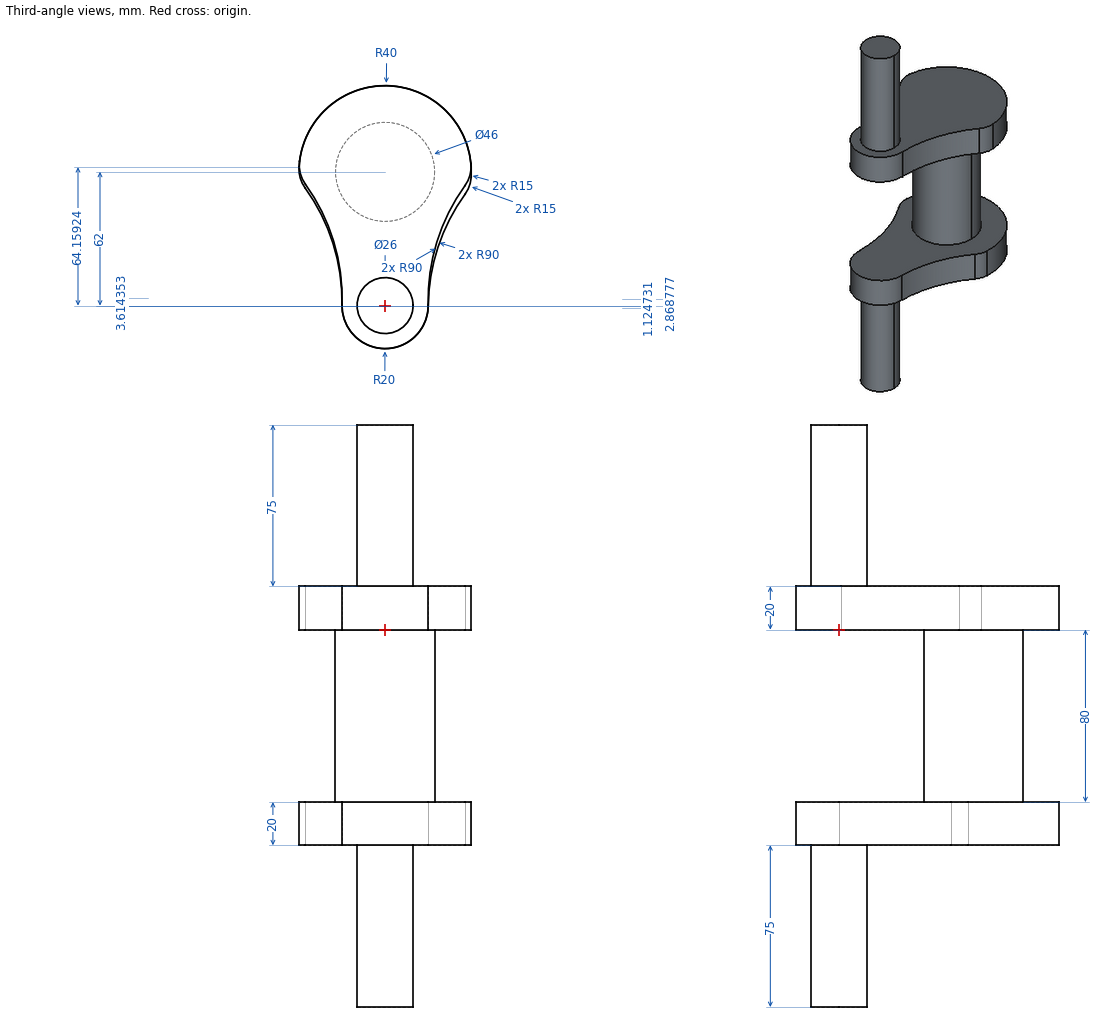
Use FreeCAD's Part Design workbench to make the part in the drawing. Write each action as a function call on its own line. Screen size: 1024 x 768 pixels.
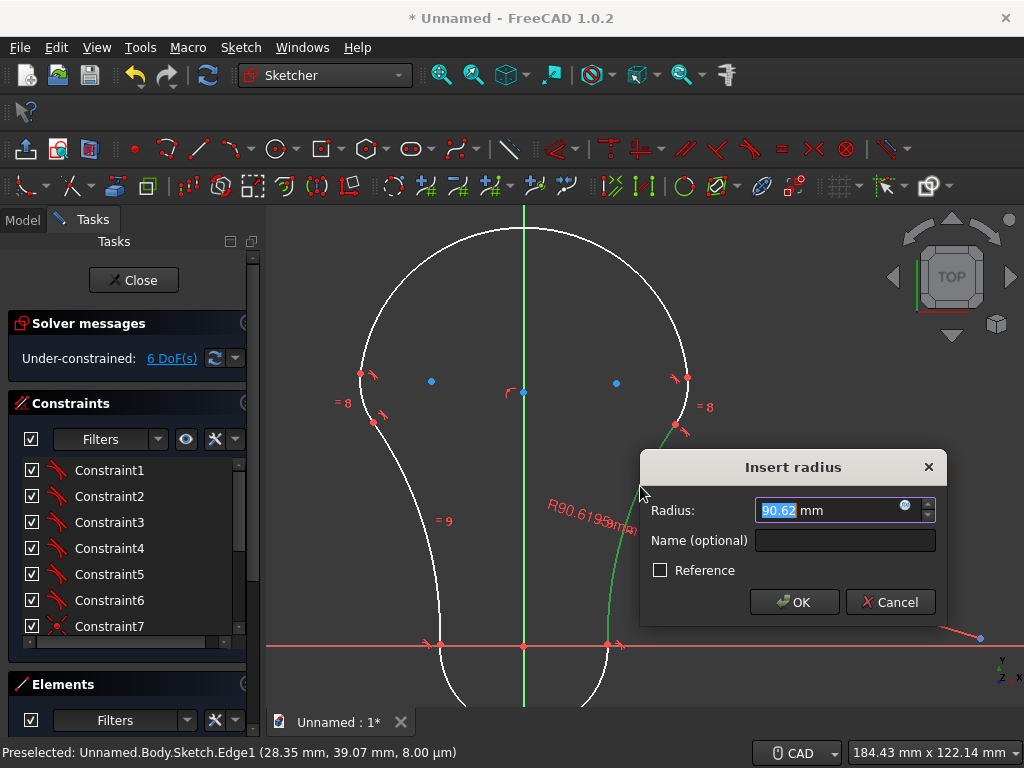
text(90)
key(Return)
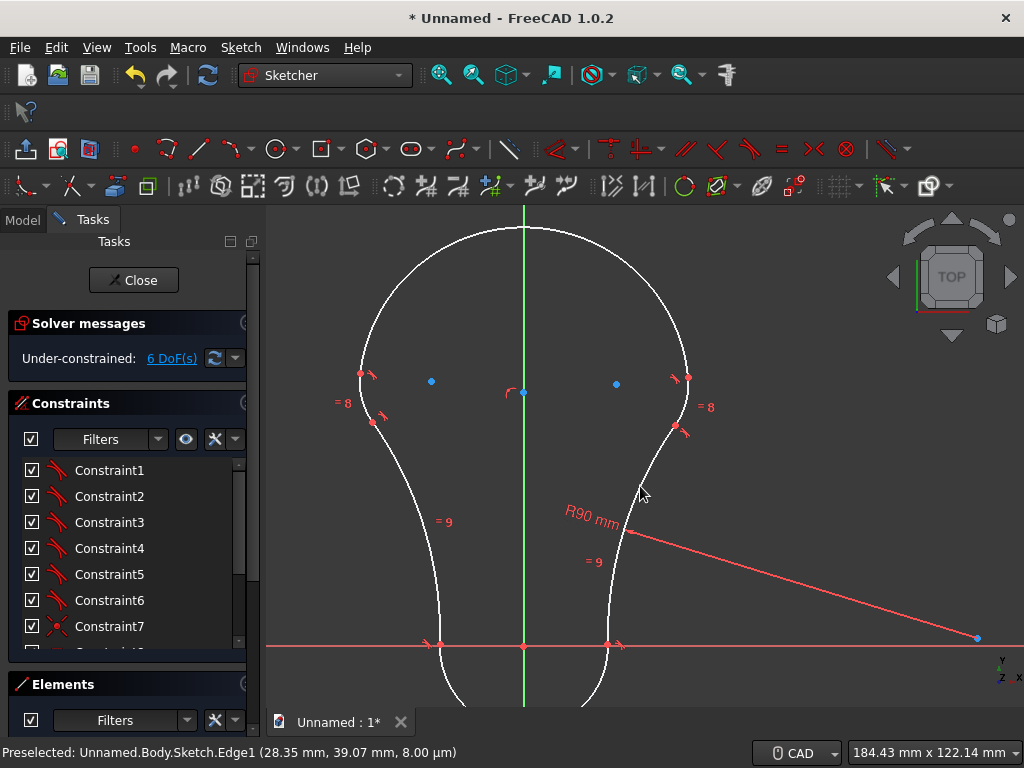
click(683, 412)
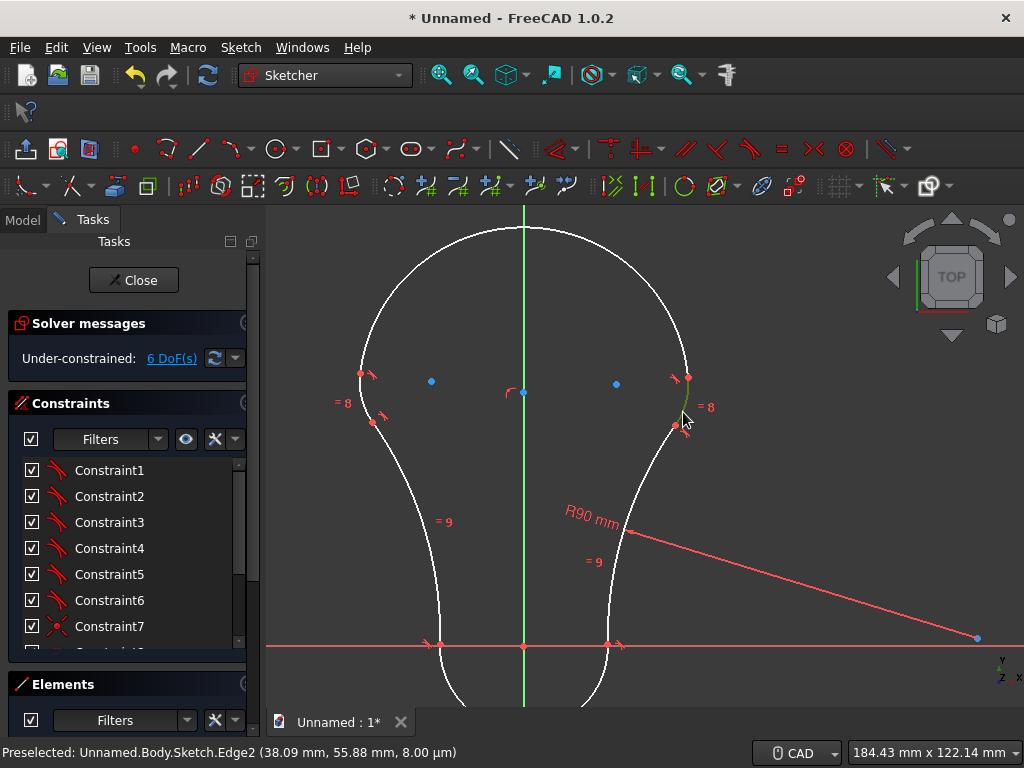
click(578, 150)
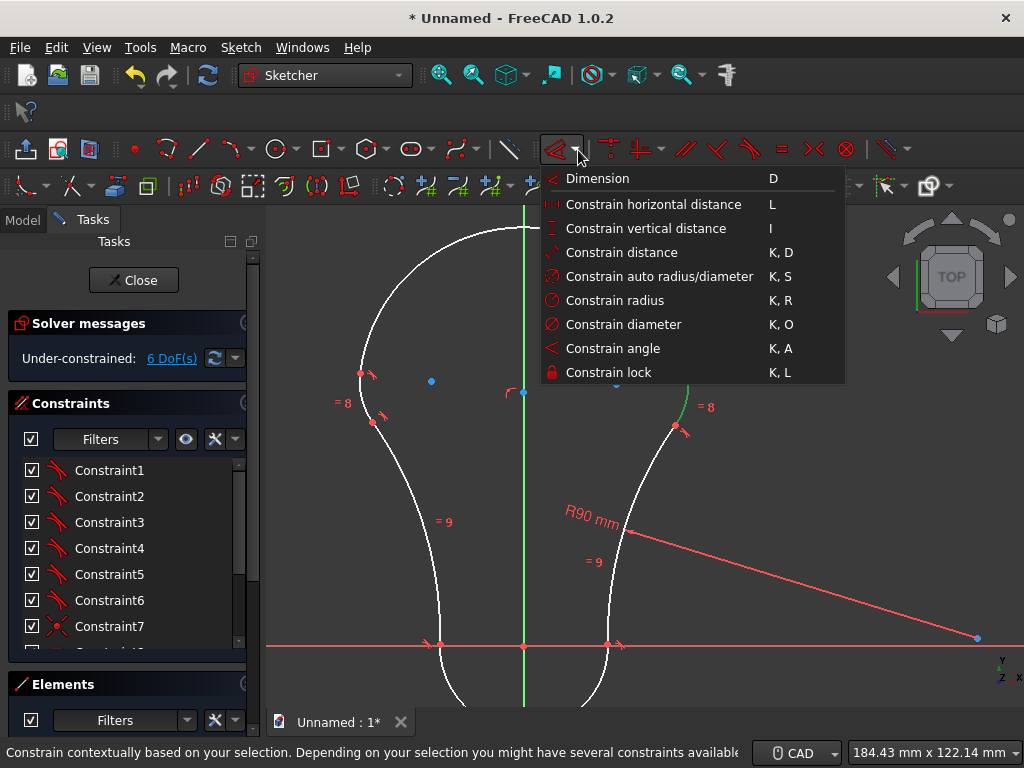
click(693, 300)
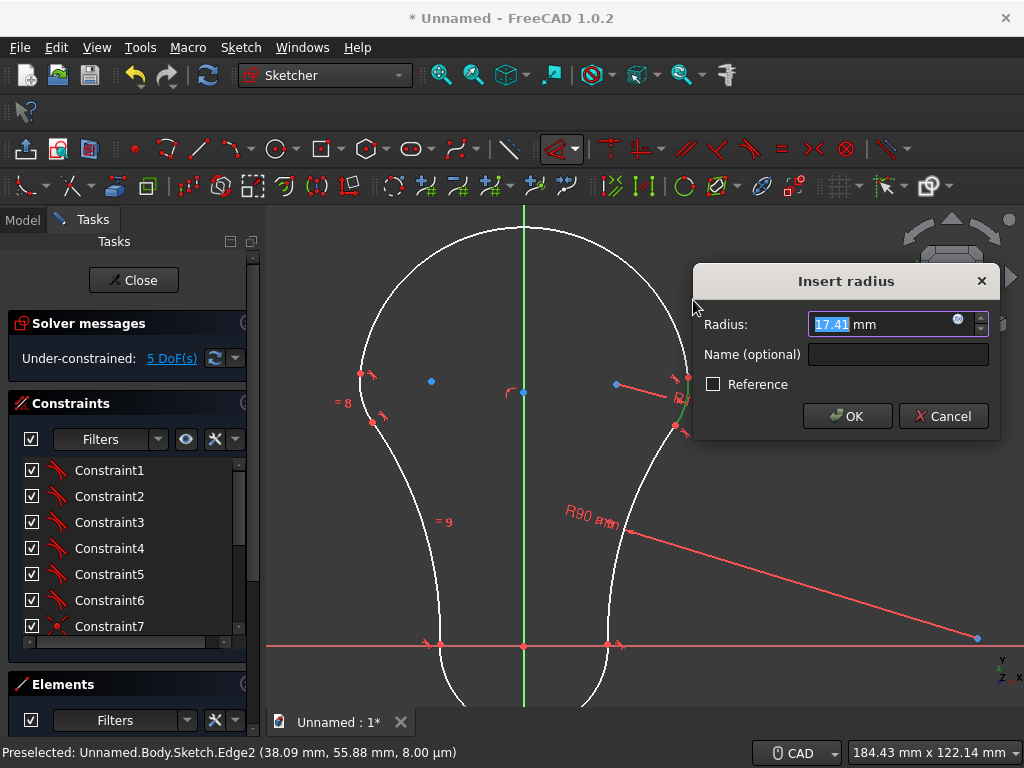
text(15)
key(Return)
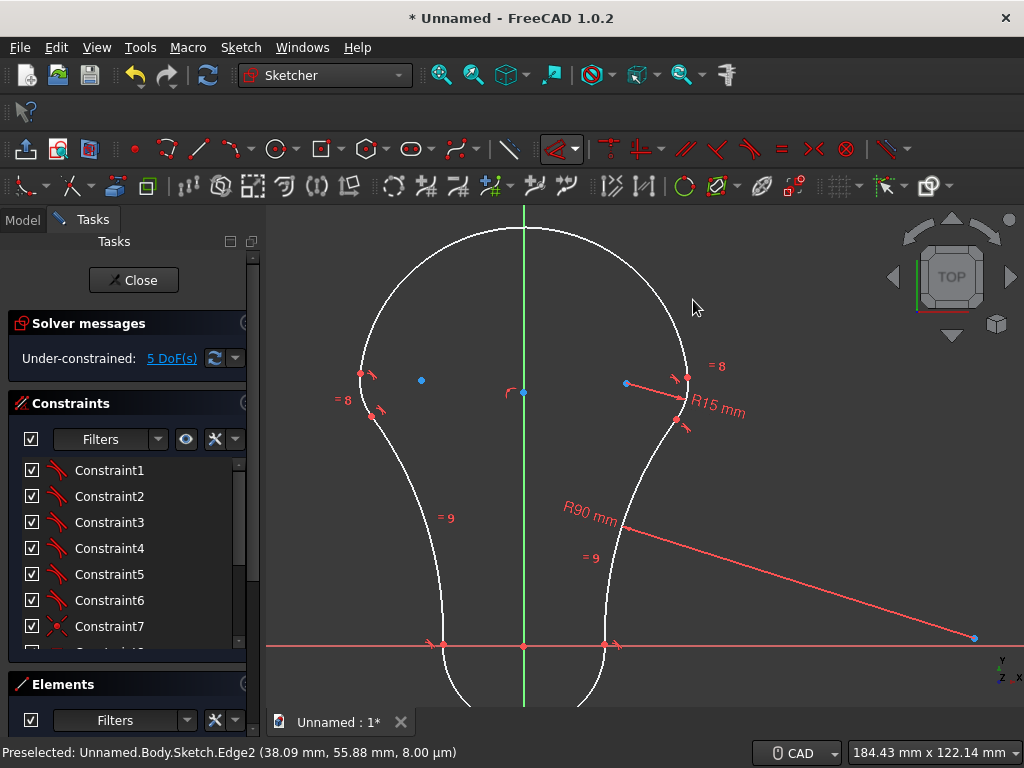
click(617, 256)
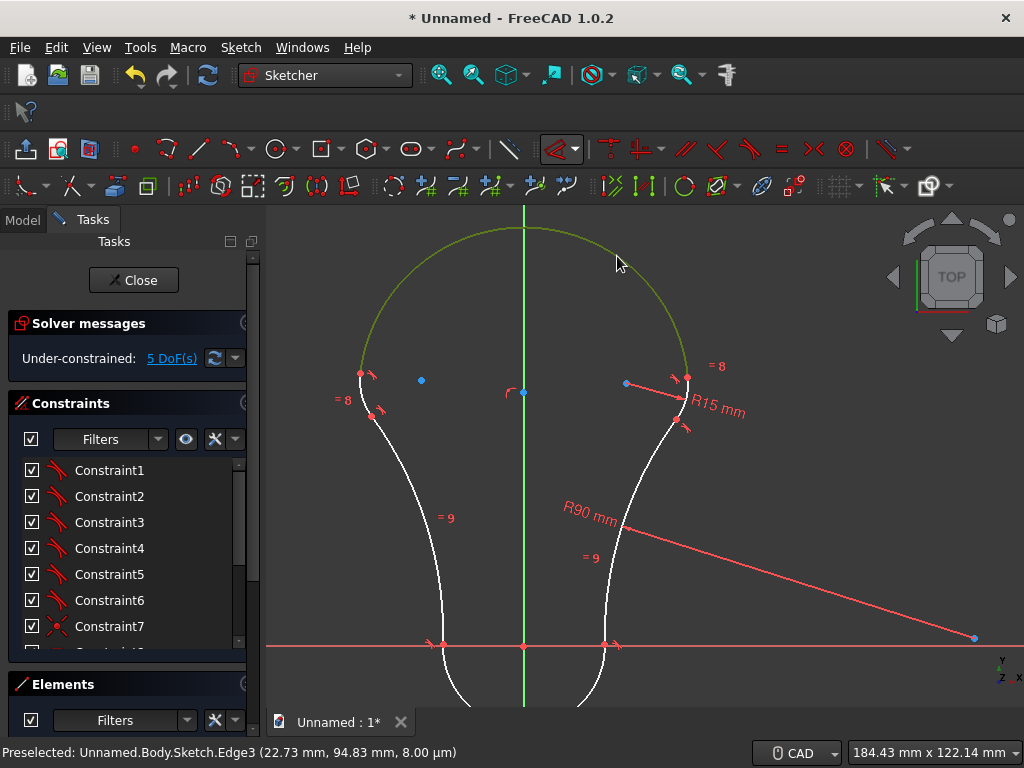
key(k)
key(r)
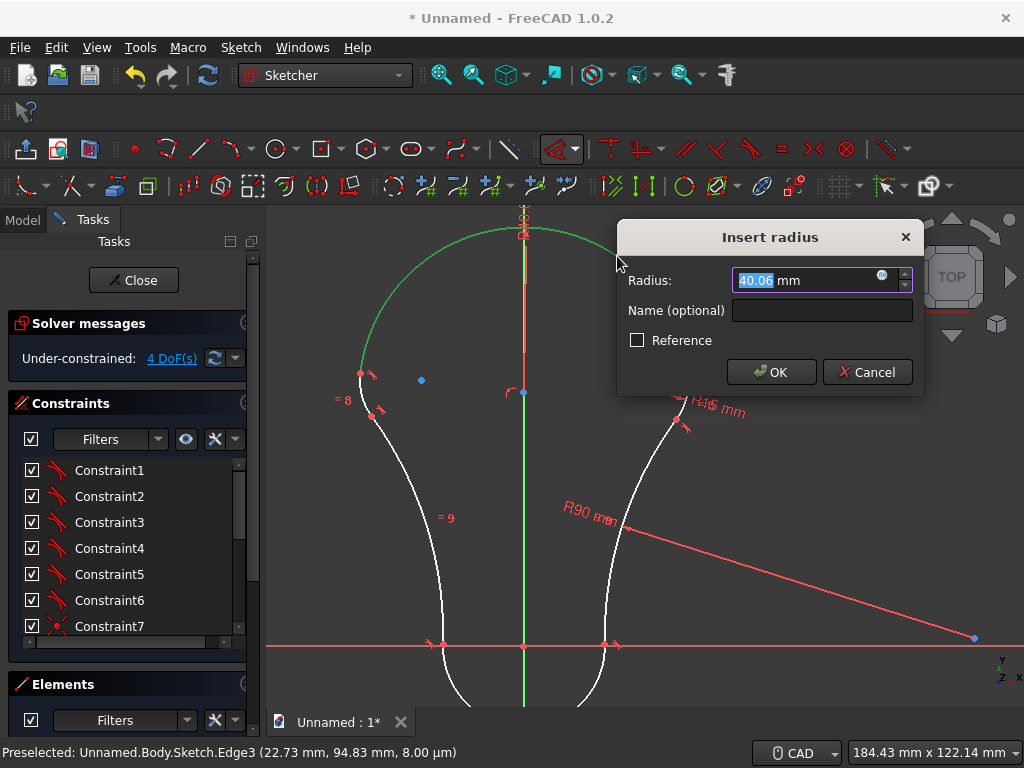
text(40)
key(Return)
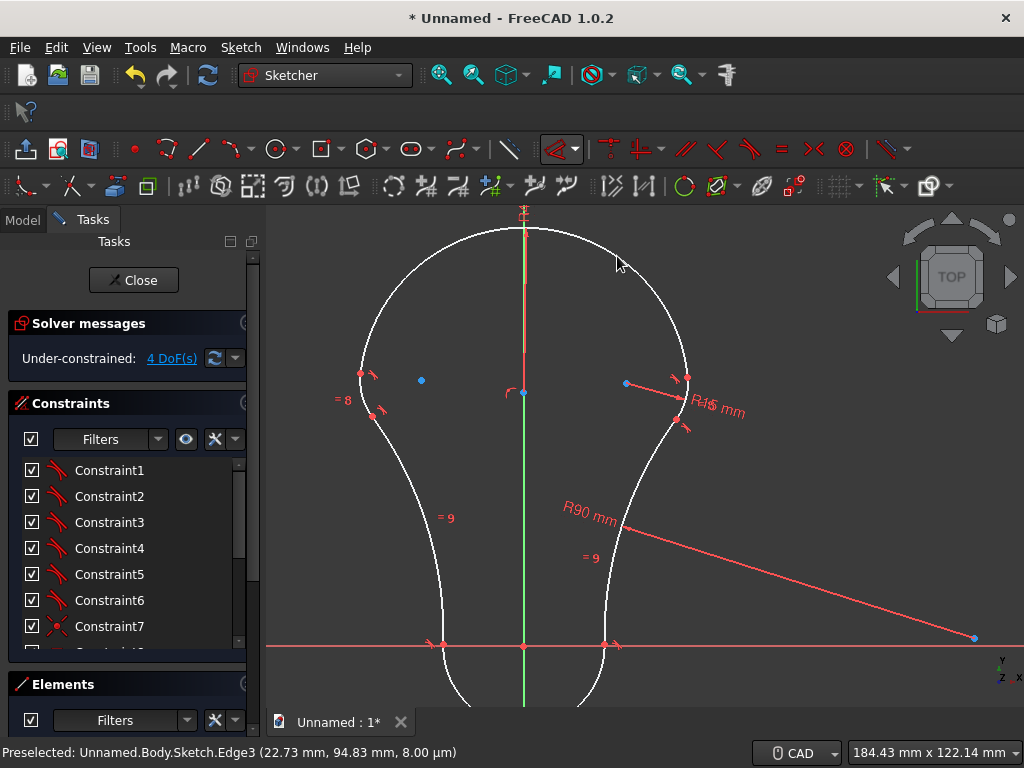
scroll(683, 412, down, 2)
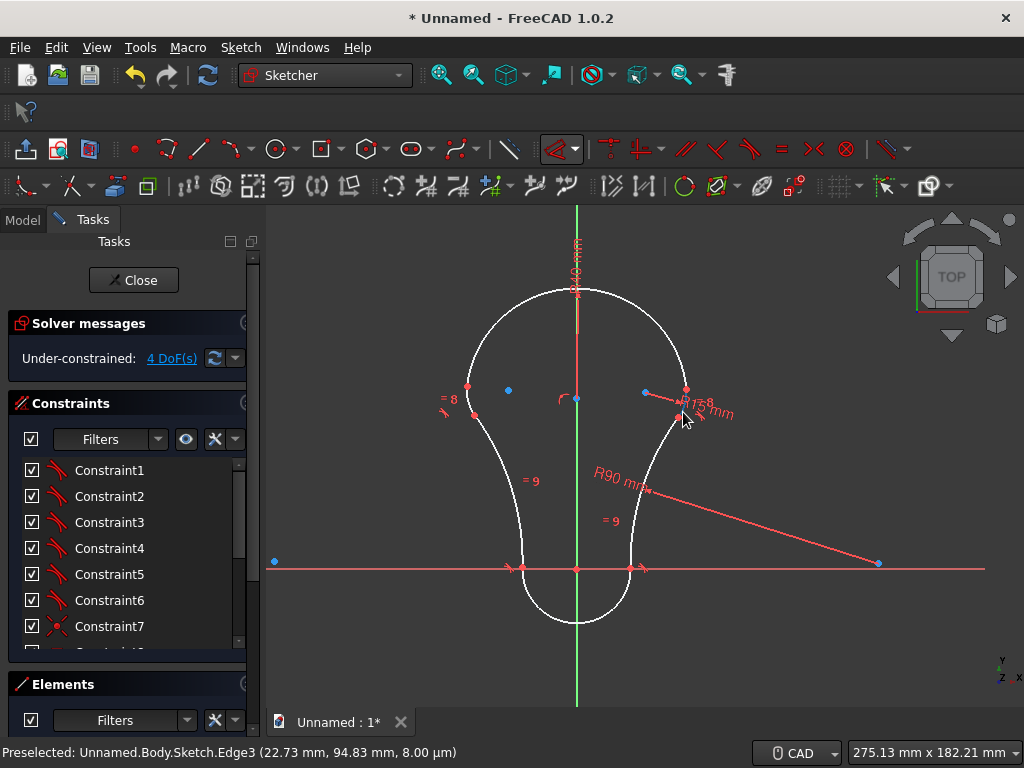
click(544, 613)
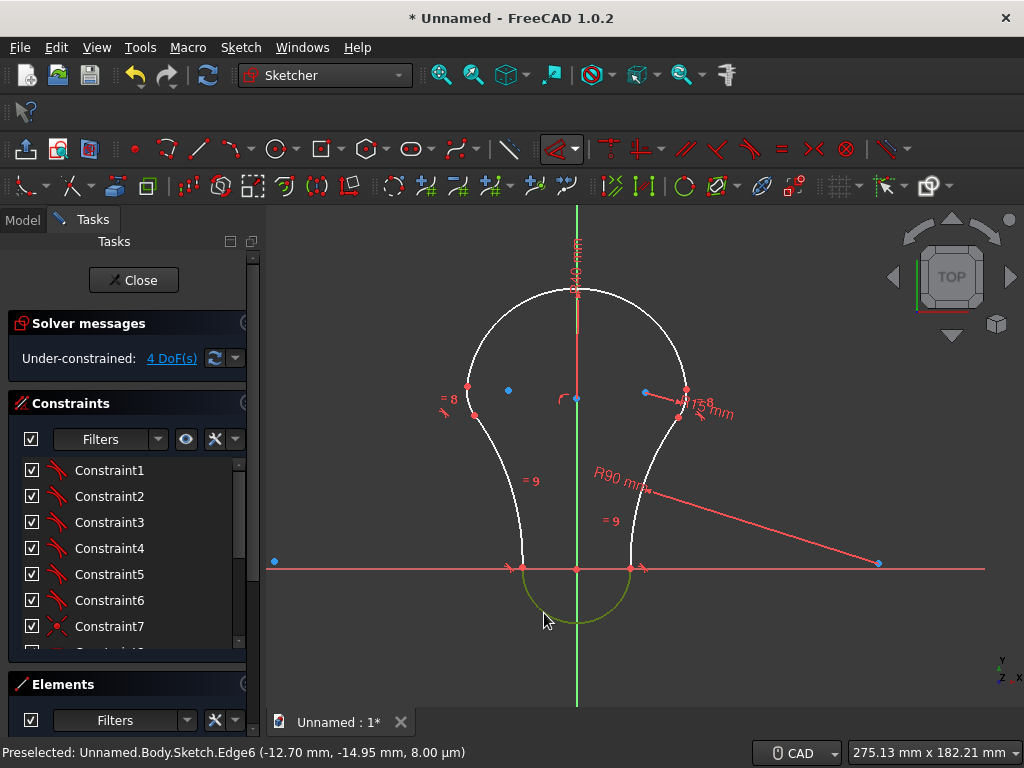
click(578, 150)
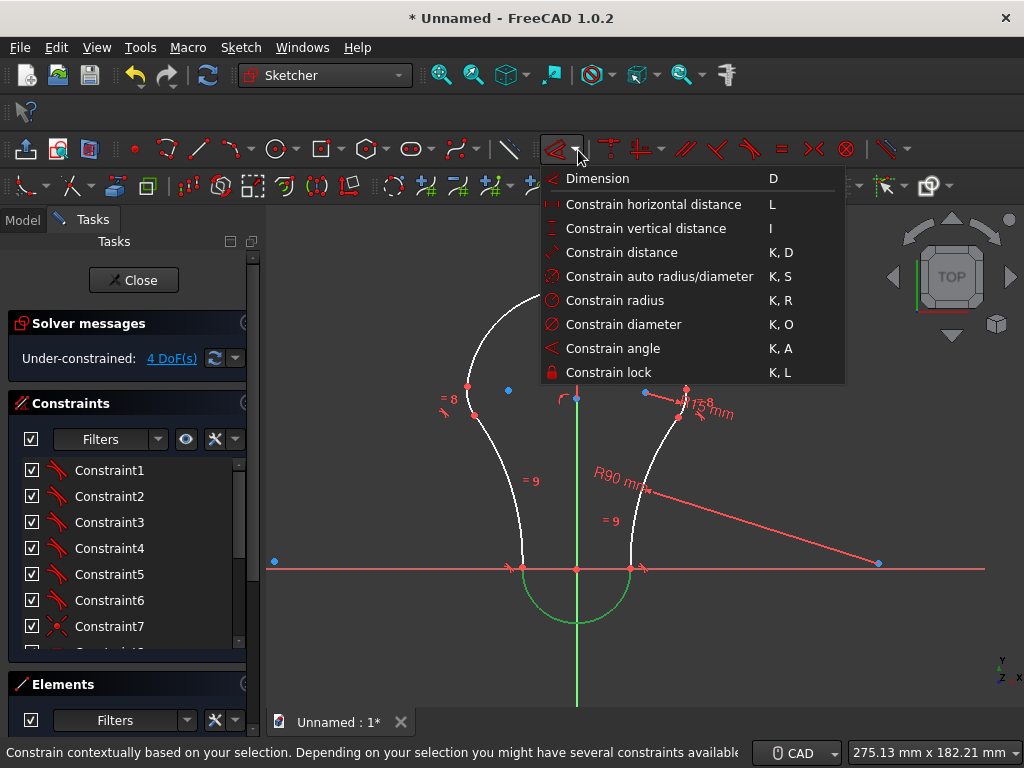
click(693, 300)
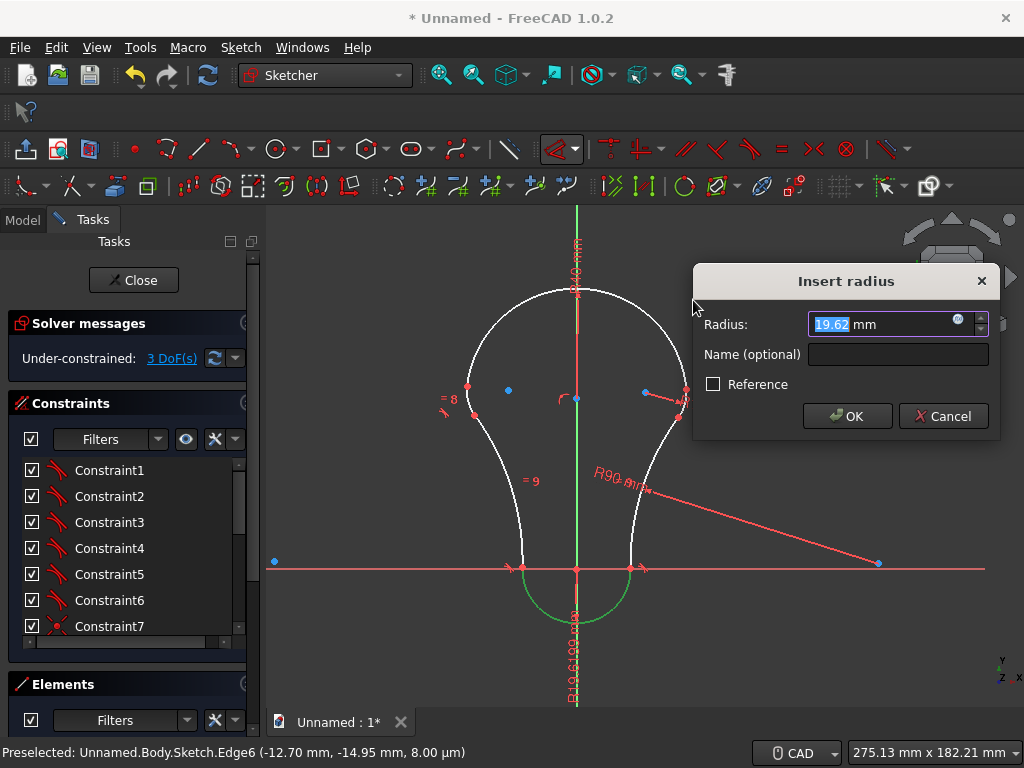
text(20)
key(Return)